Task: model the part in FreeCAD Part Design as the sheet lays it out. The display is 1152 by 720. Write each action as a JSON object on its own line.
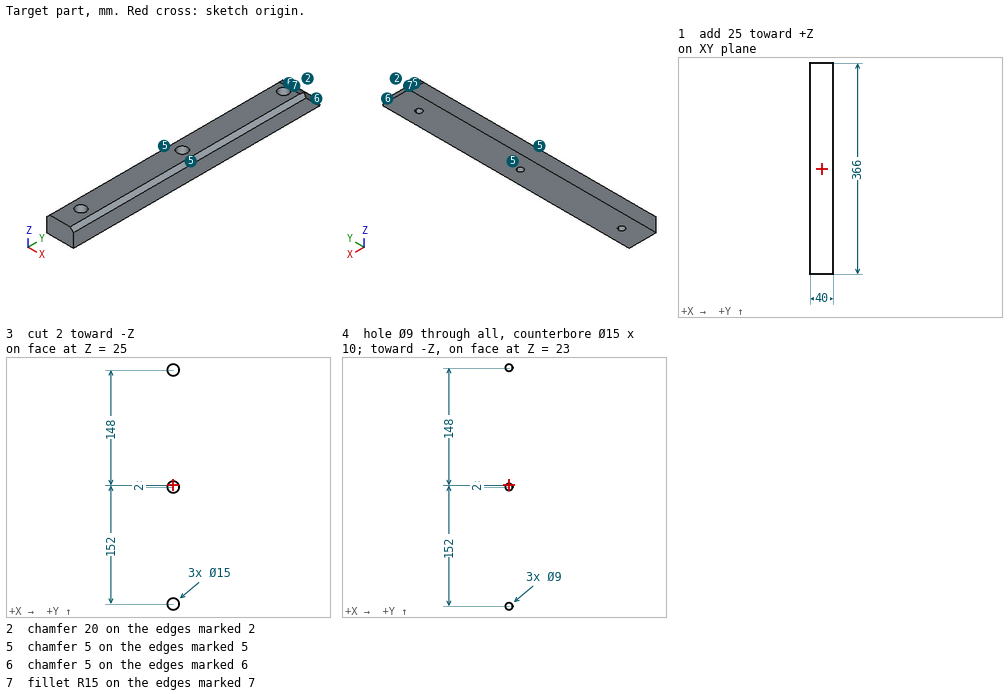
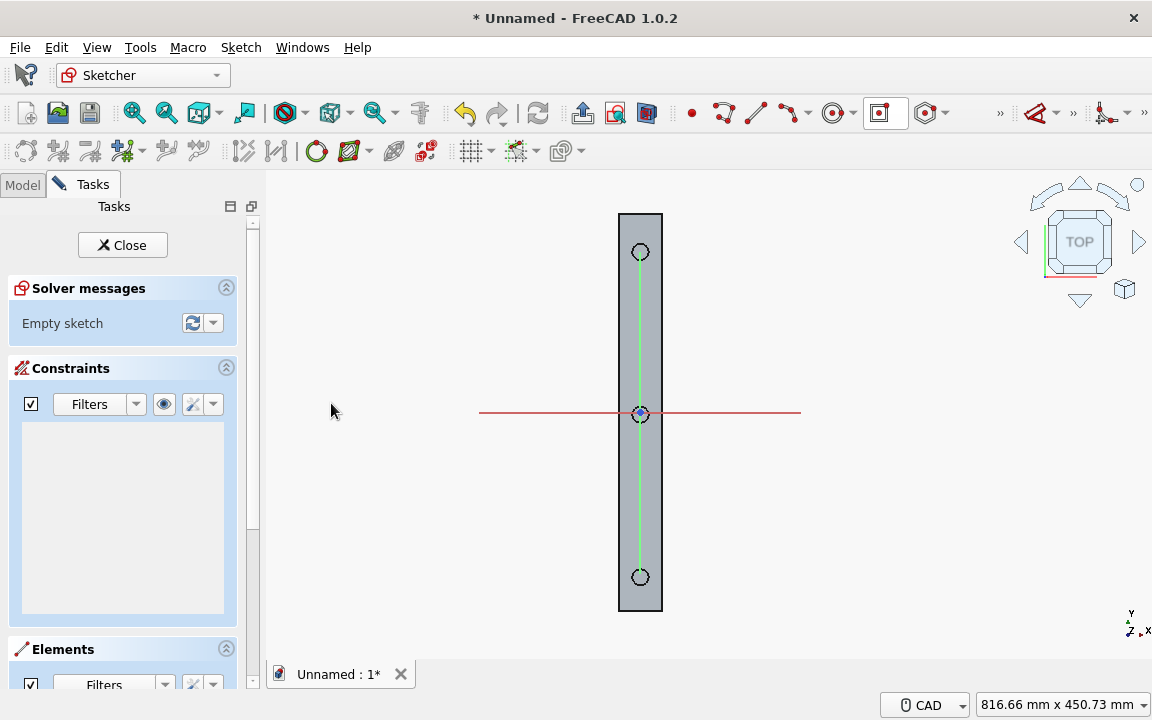
{"action": "left_click", "coordinate": [834, 114]}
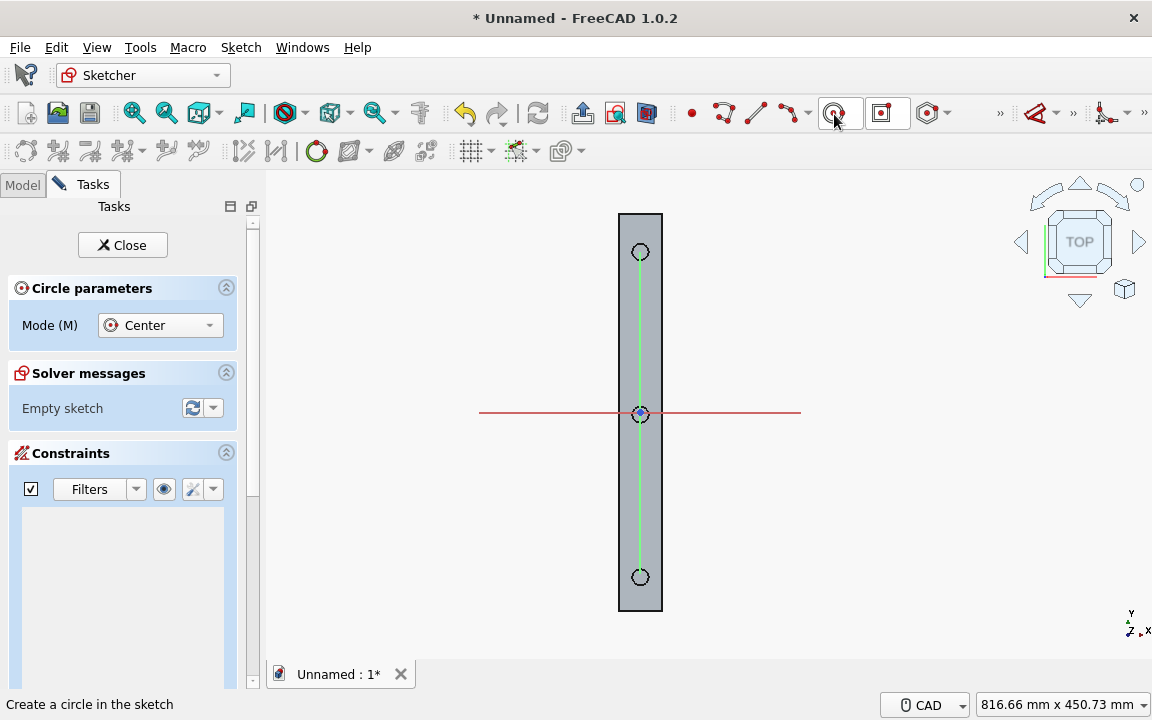
{"action": "scroll", "coordinate": [640, 577], "scroll_direction": "up", "scroll_amount": 8}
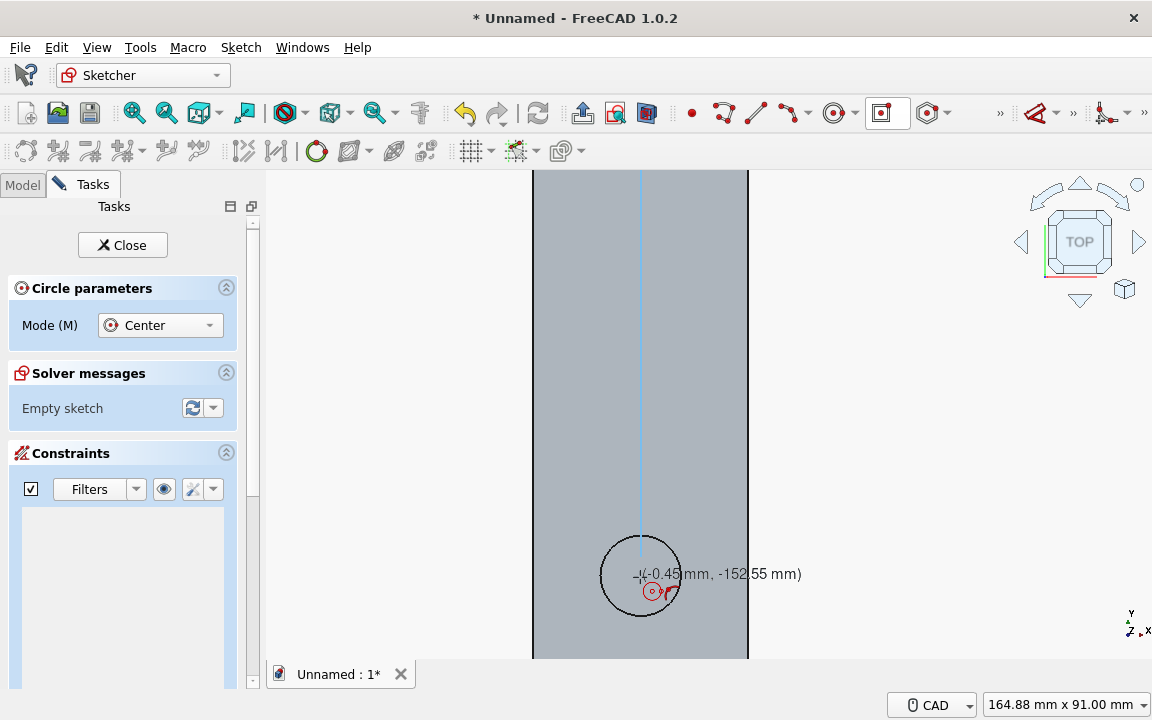
{"action": "scroll", "coordinate": [640, 578], "scroll_direction": "down", "scroll_amount": 8}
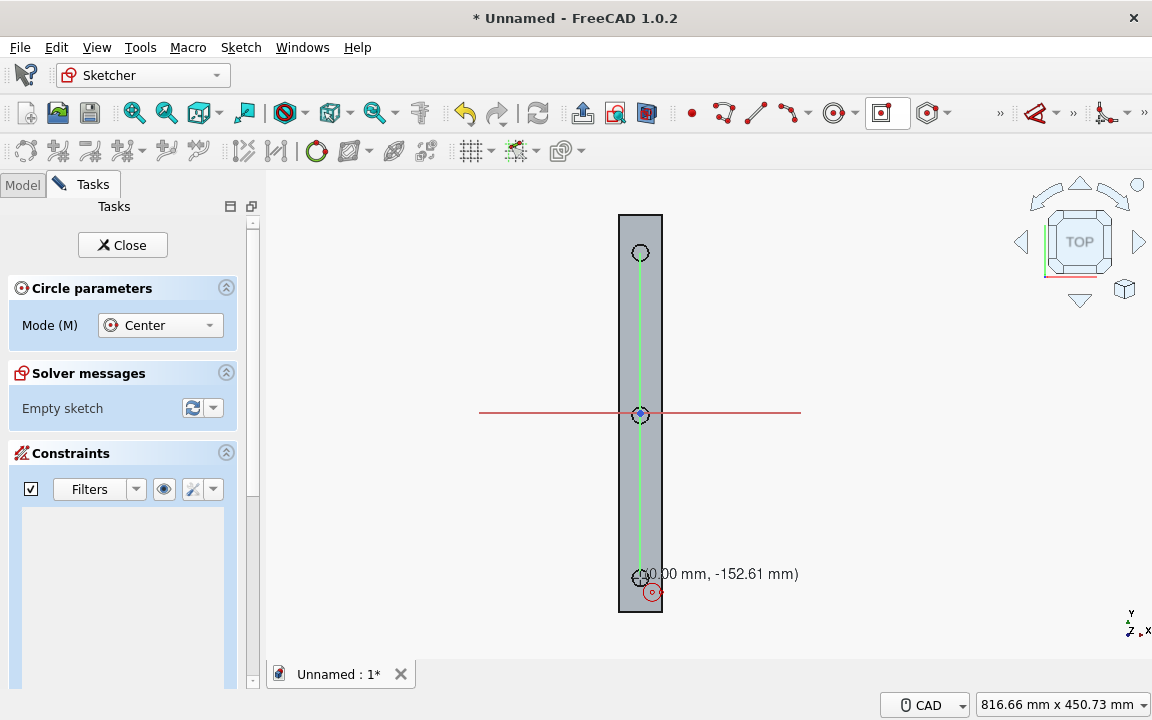
{"action": "left_click", "coordinate": [640, 578]}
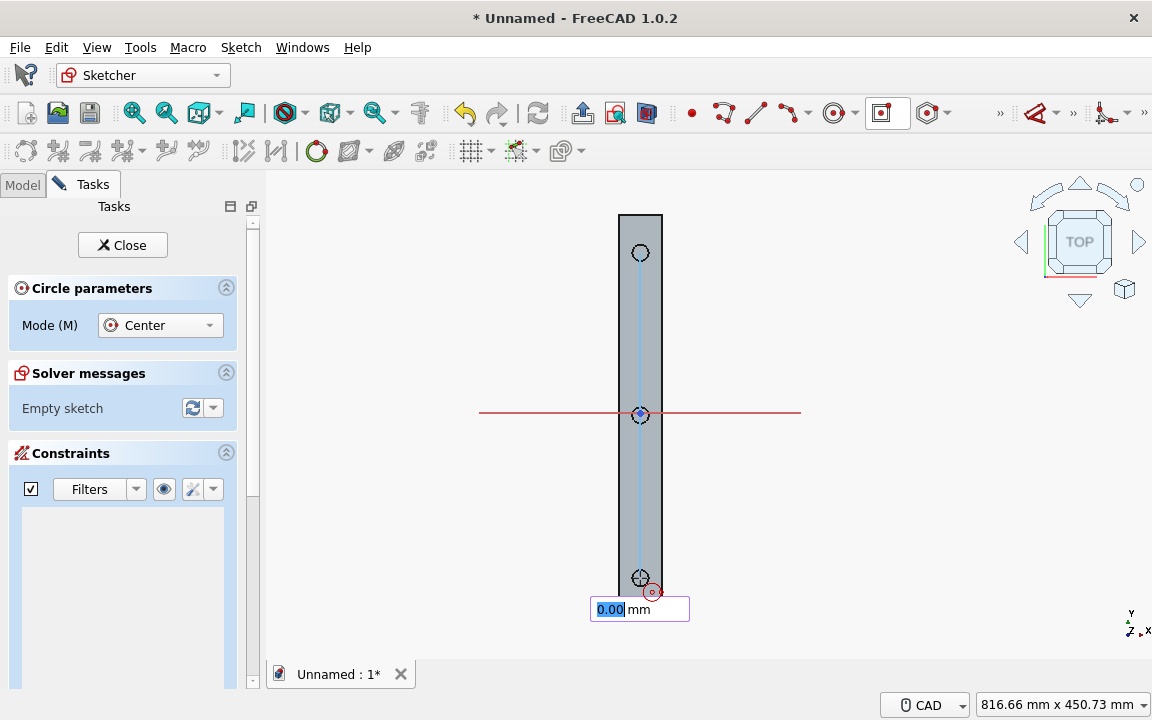
{"action": "scroll", "coordinate": [645, 577], "scroll_direction": "up", "scroll_amount": 7}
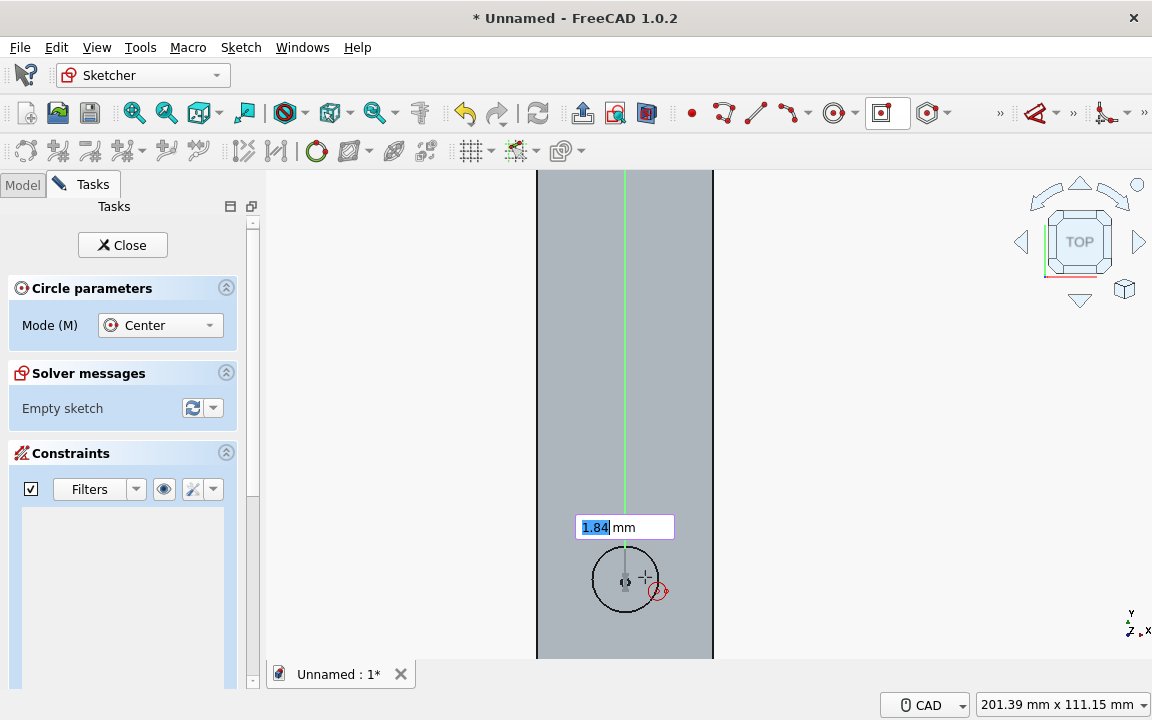
{"action": "left_click", "coordinate": [644, 573]}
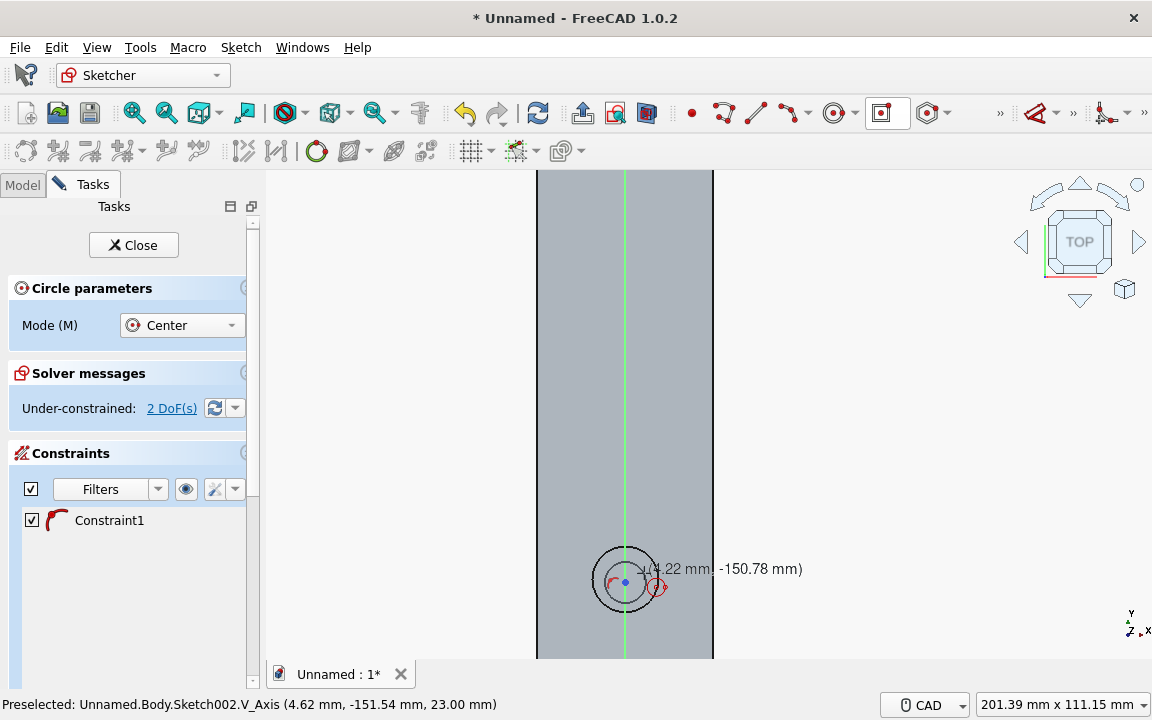
{"action": "scroll", "coordinate": [645, 577], "scroll_direction": "down", "scroll_amount": 7}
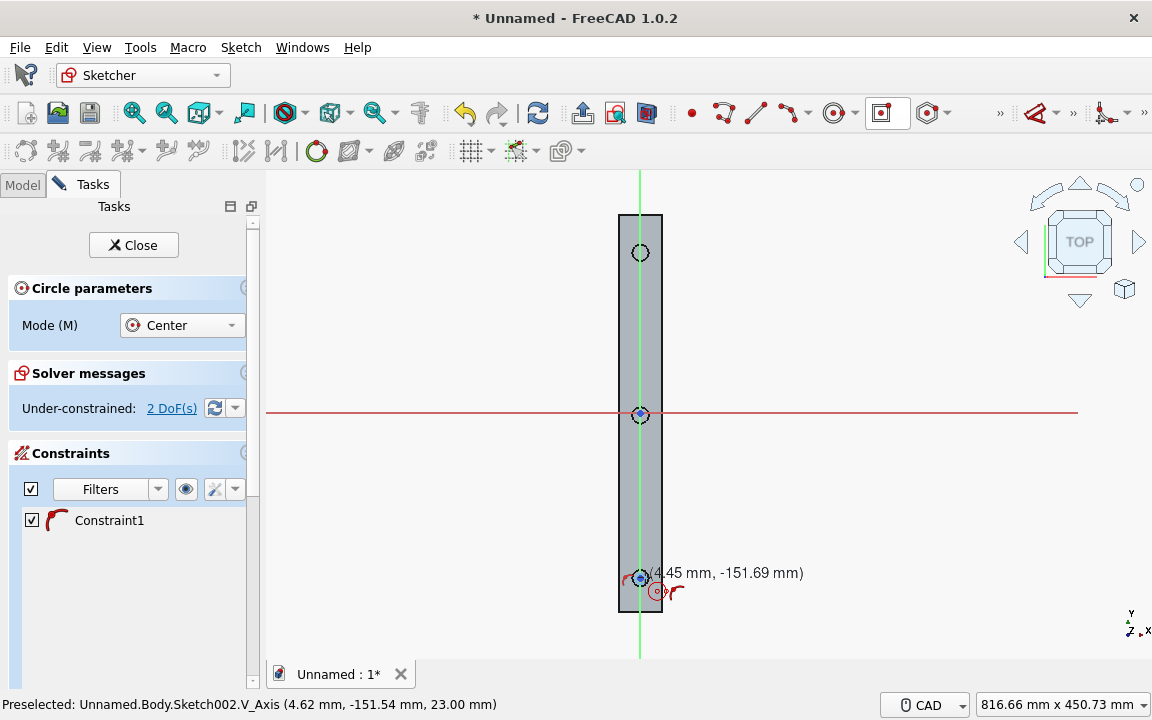
{"action": "scroll", "coordinate": [640, 415], "scroll_direction": "up", "scroll_amount": 10}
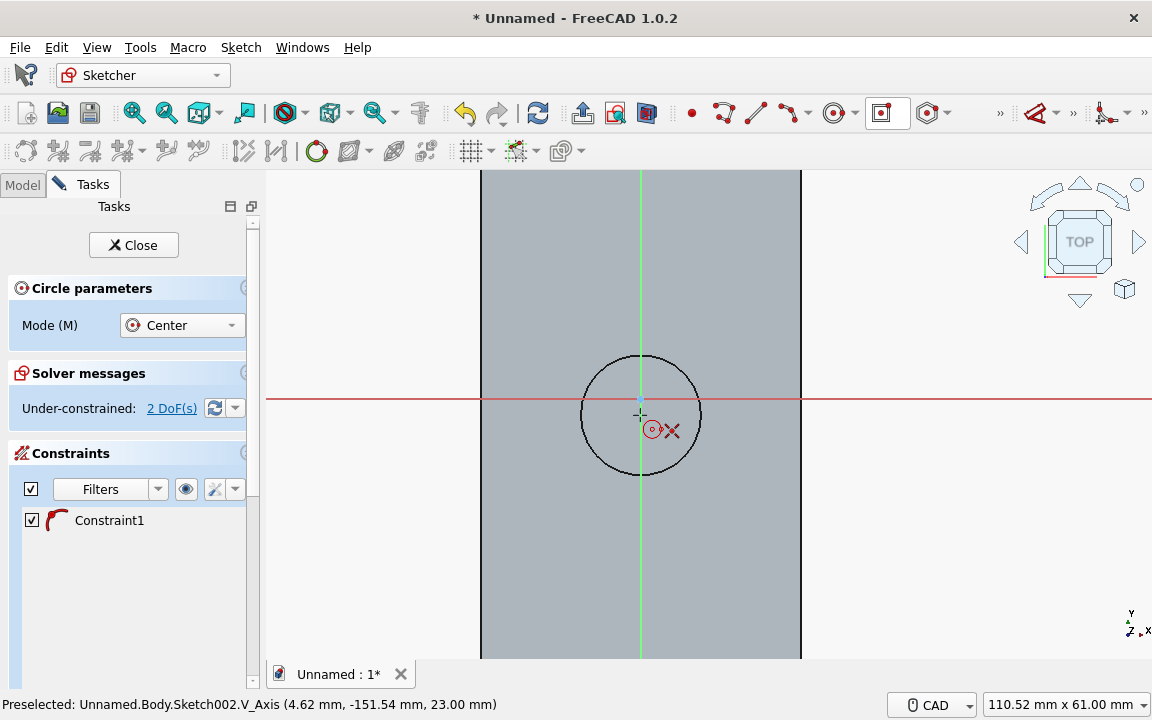
{"action": "left_click", "coordinate": [641, 415]}
{"action": "left_click", "coordinate": [666, 441]}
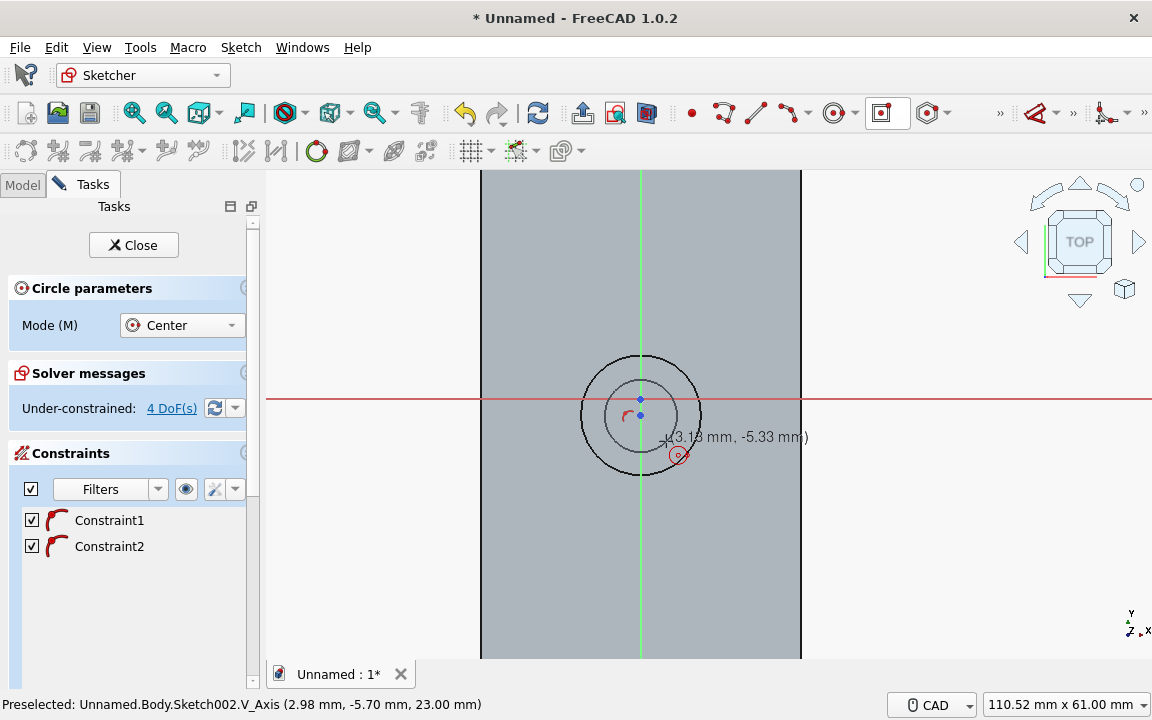
{"action": "scroll", "coordinate": [640, 414], "scroll_direction": "down", "scroll_amount": 10}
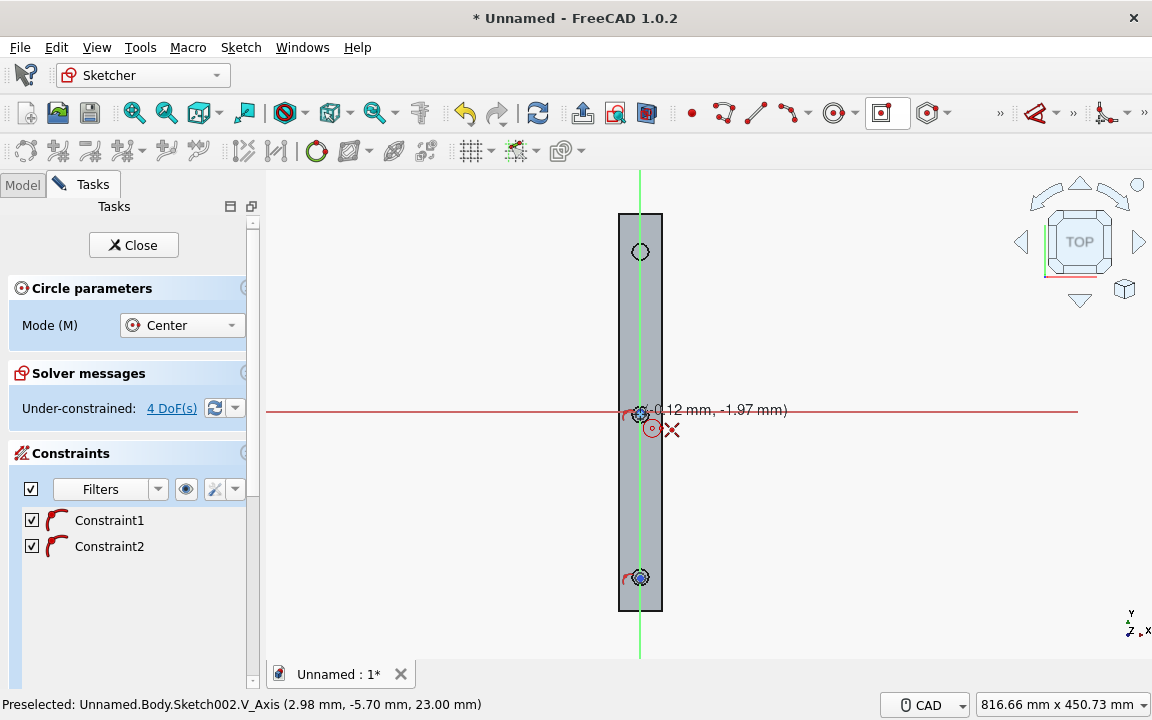
{"action": "scroll", "coordinate": [640, 252], "scroll_direction": "up", "scroll_amount": 8}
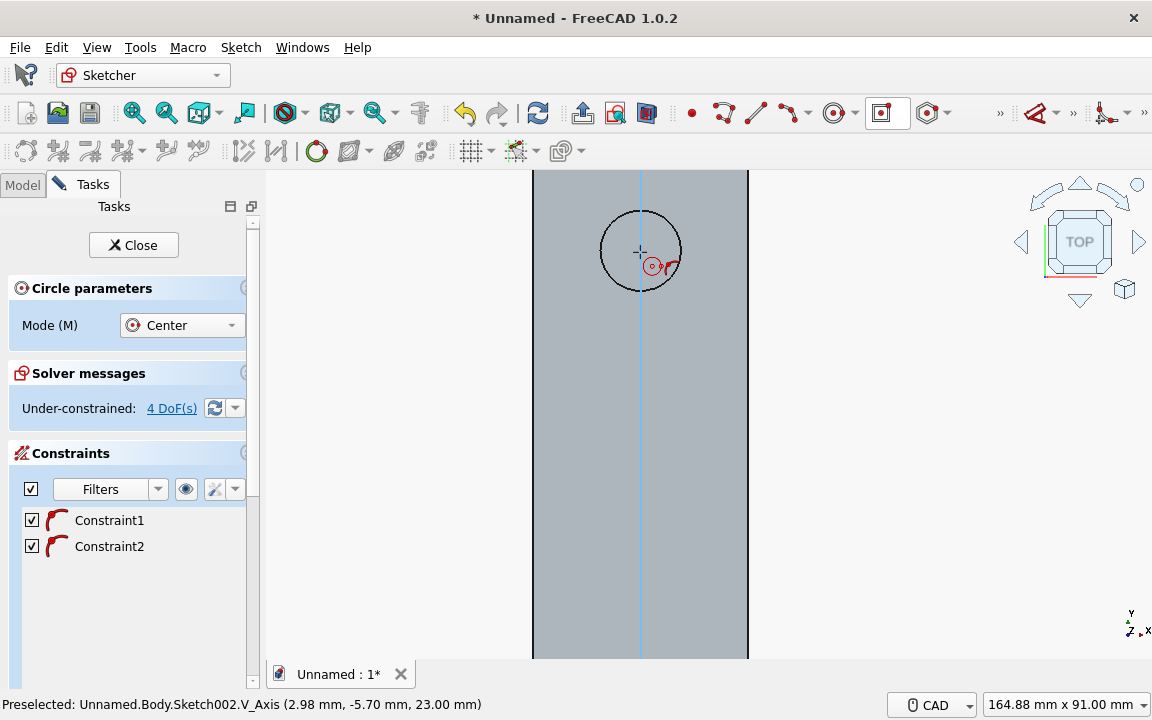
{"action": "scroll", "coordinate": [640, 252], "scroll_direction": "down", "scroll_amount": 8}